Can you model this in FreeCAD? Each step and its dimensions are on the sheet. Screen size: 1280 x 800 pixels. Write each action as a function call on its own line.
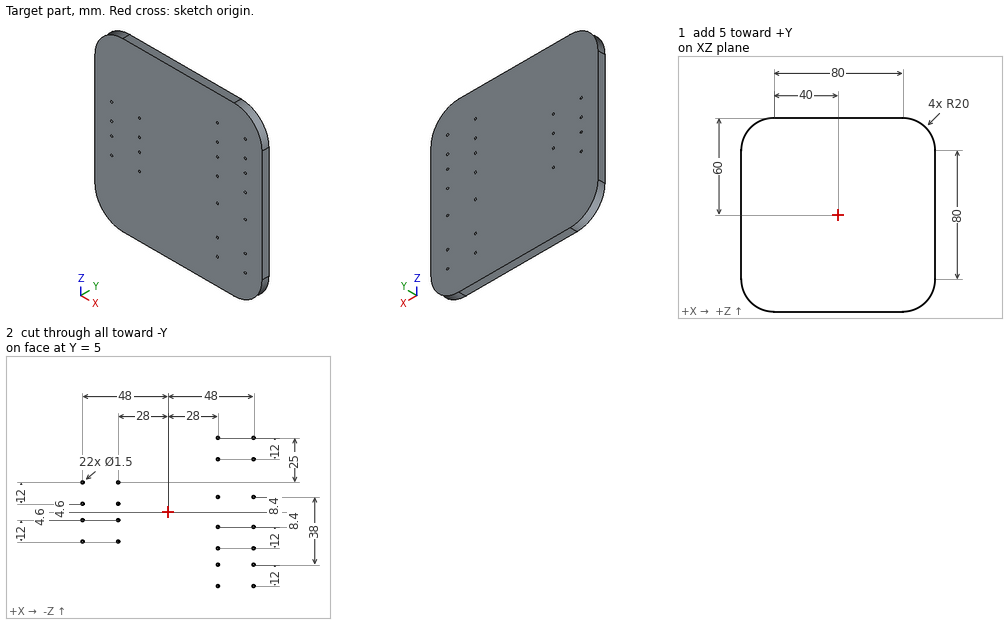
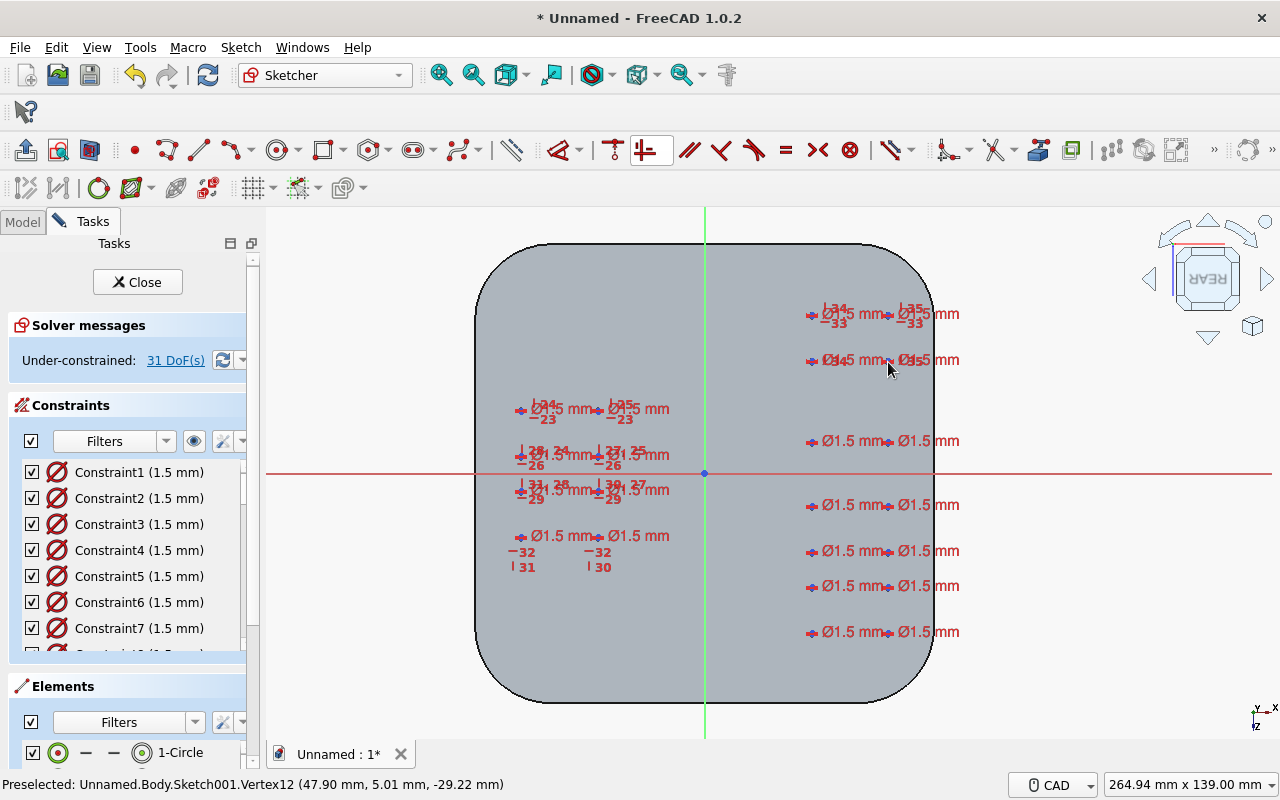
click(812, 362)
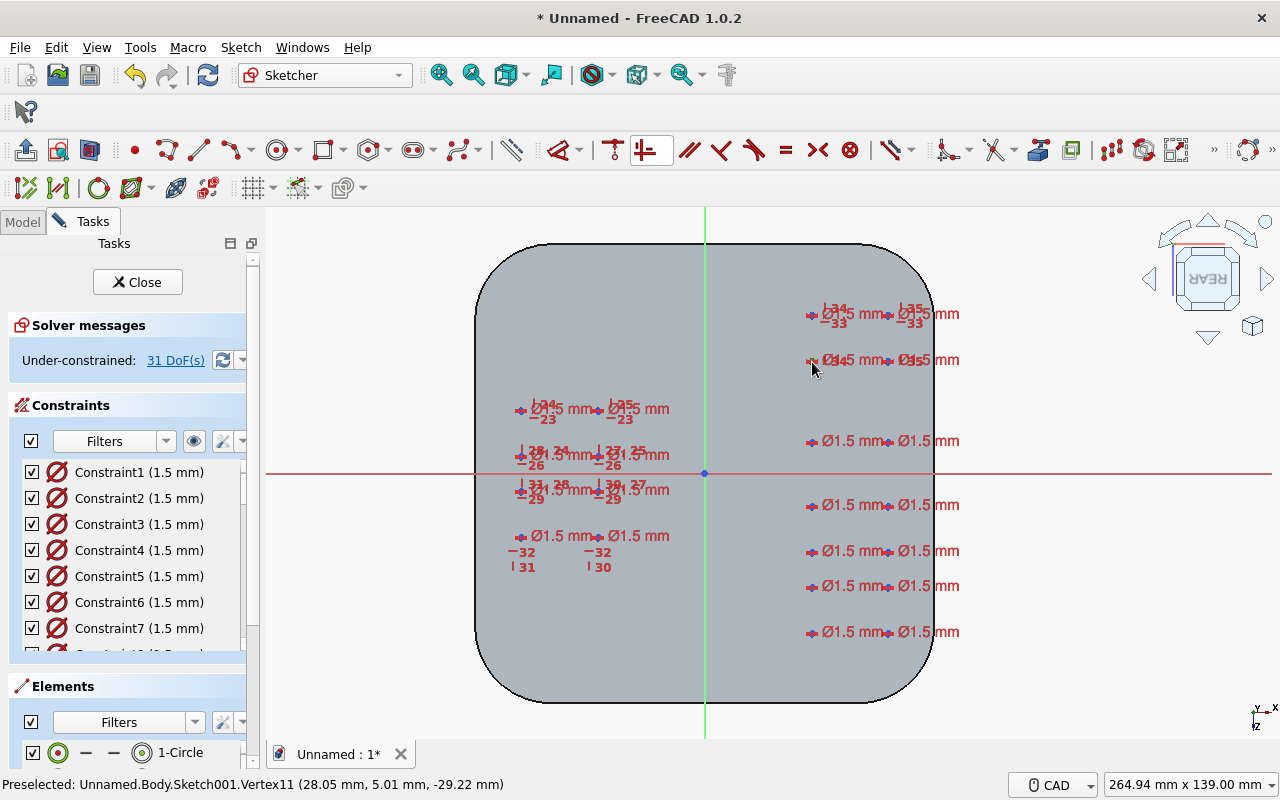
click(888, 362)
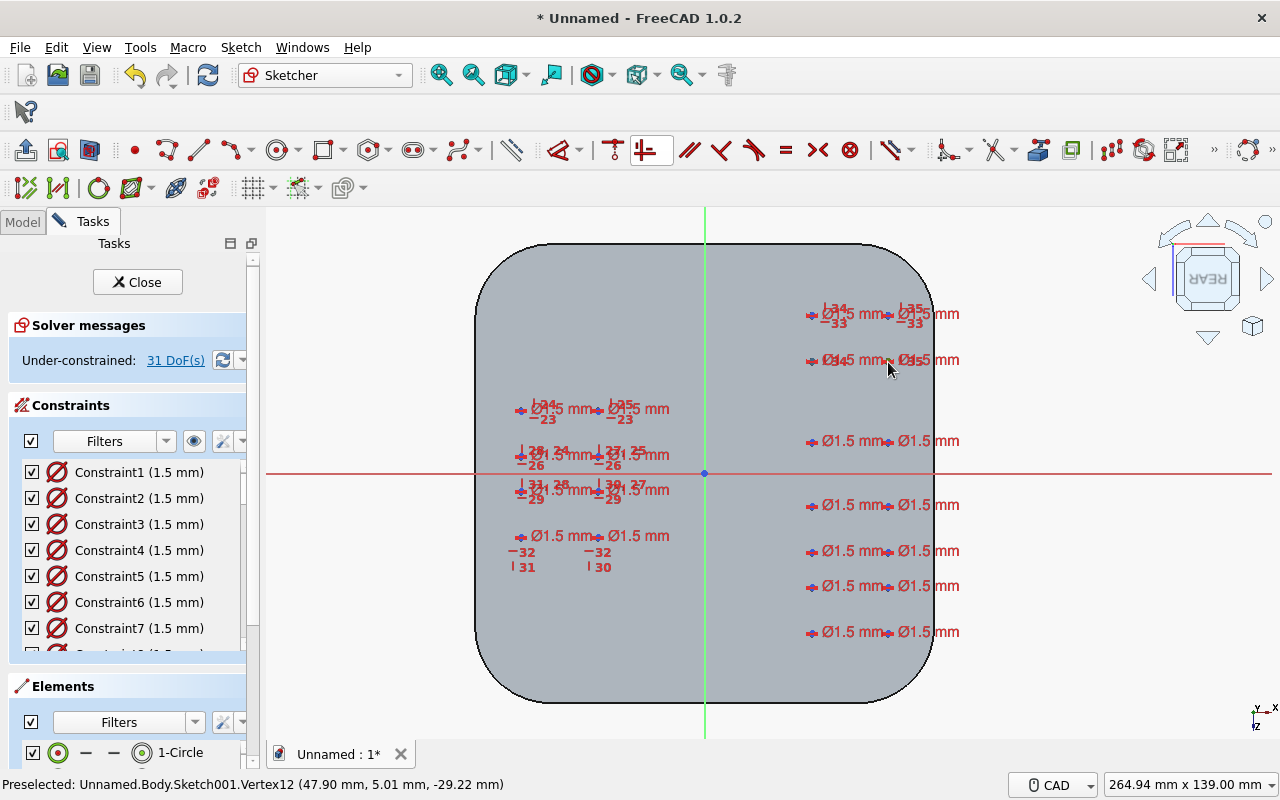
click(668, 150)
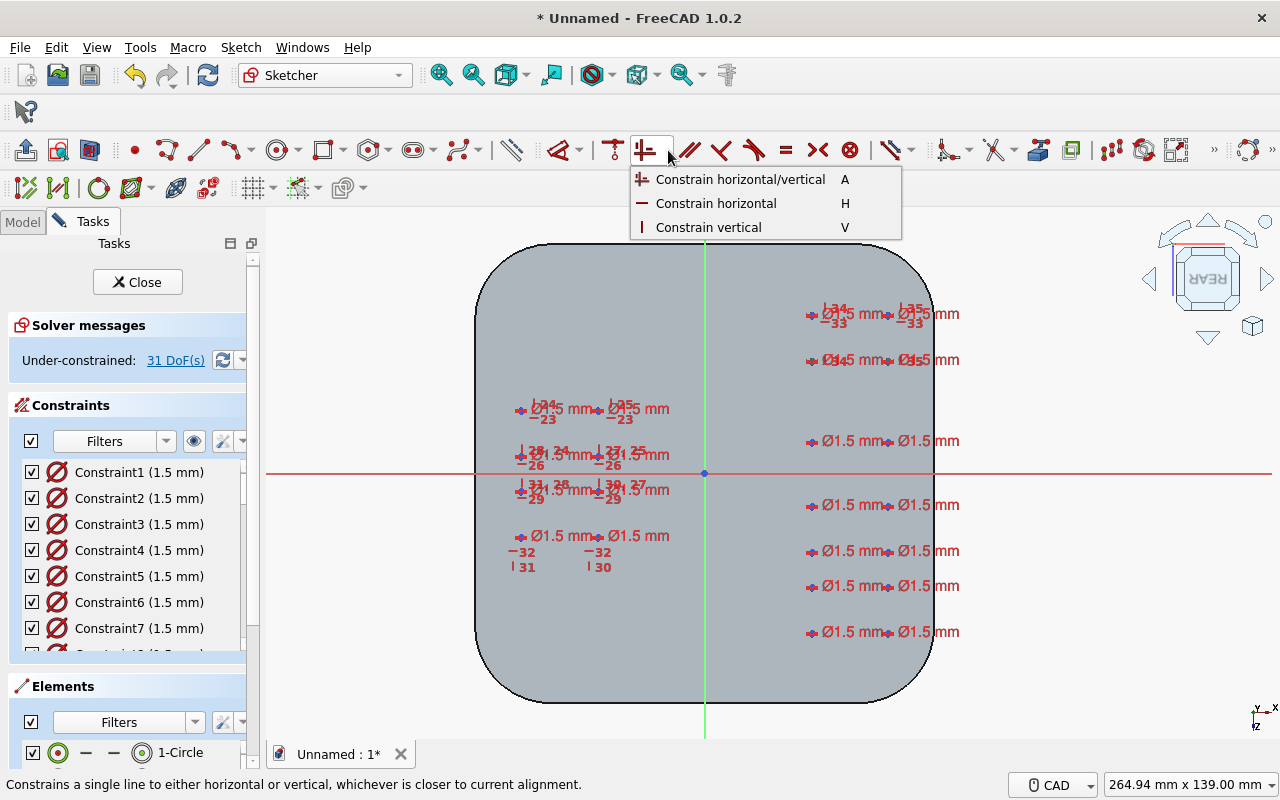
click(766, 203)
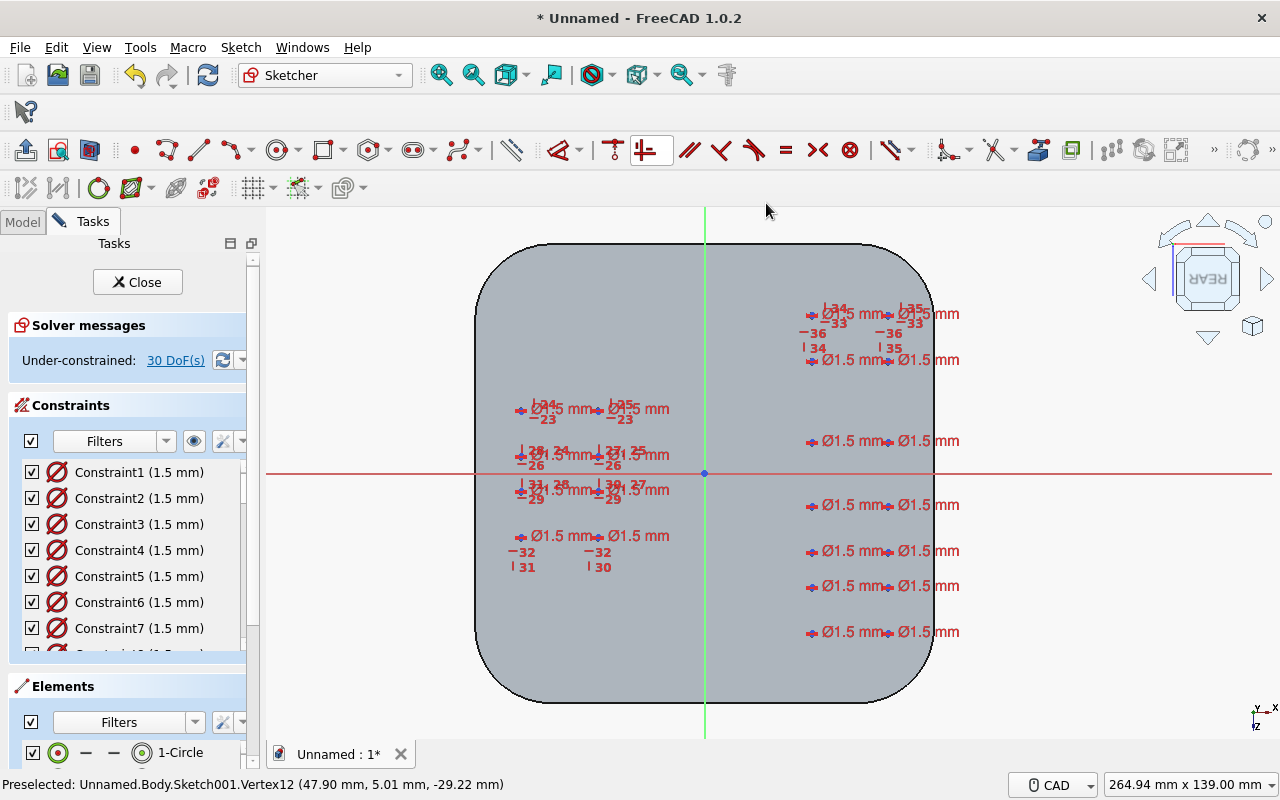
click(888, 362)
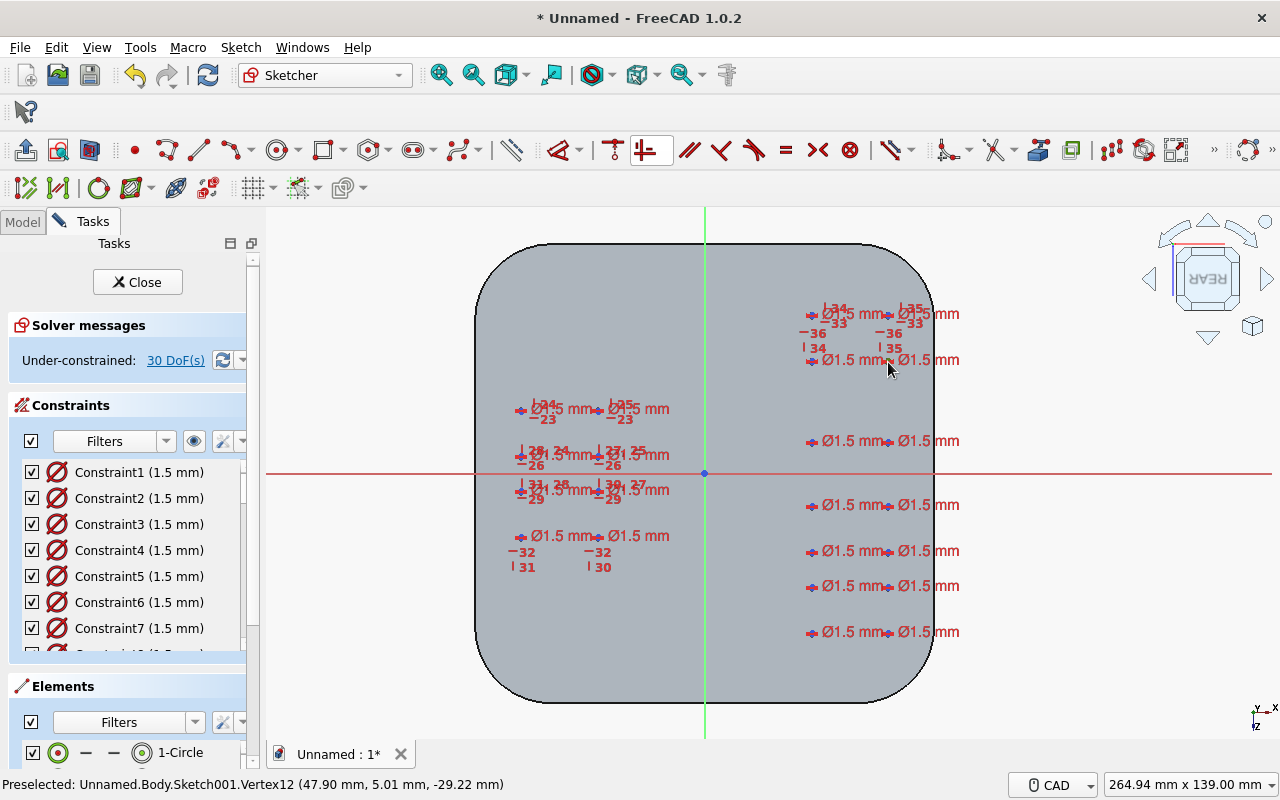
click(888, 443)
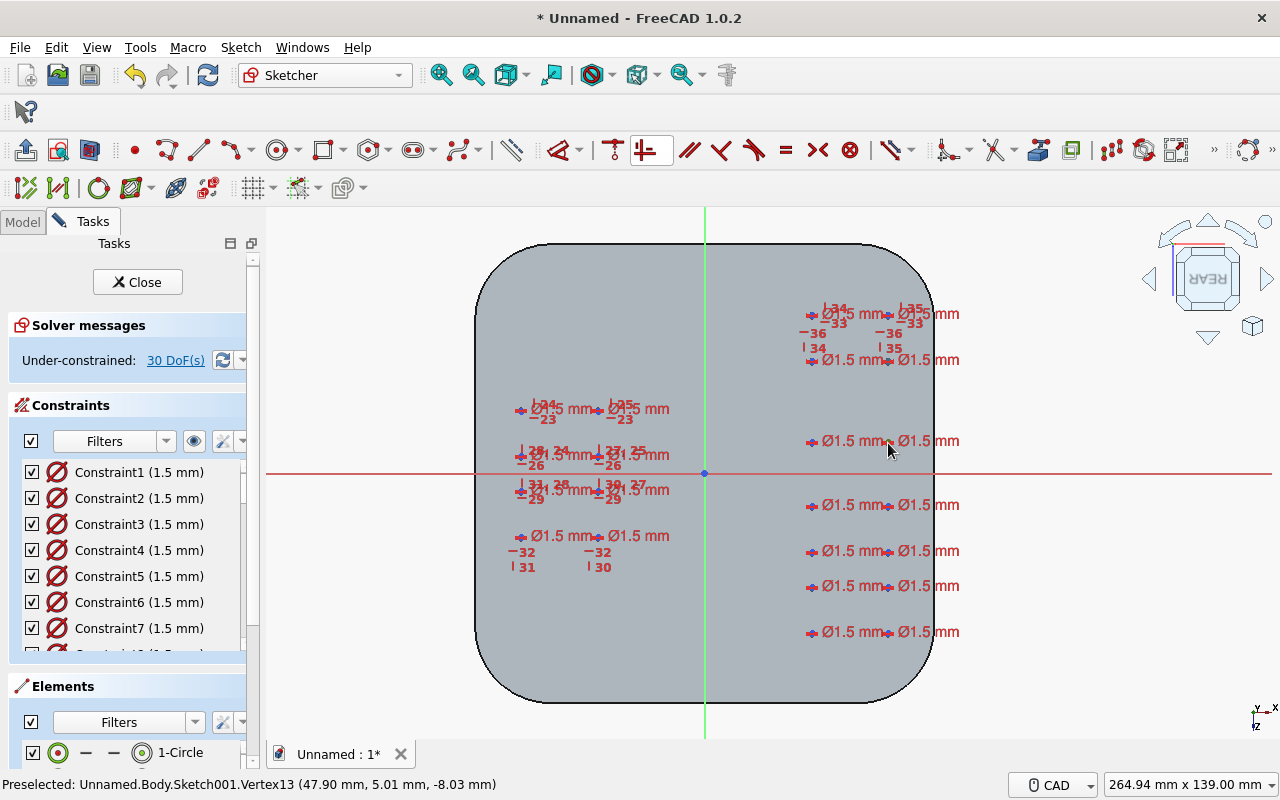
click(668, 150)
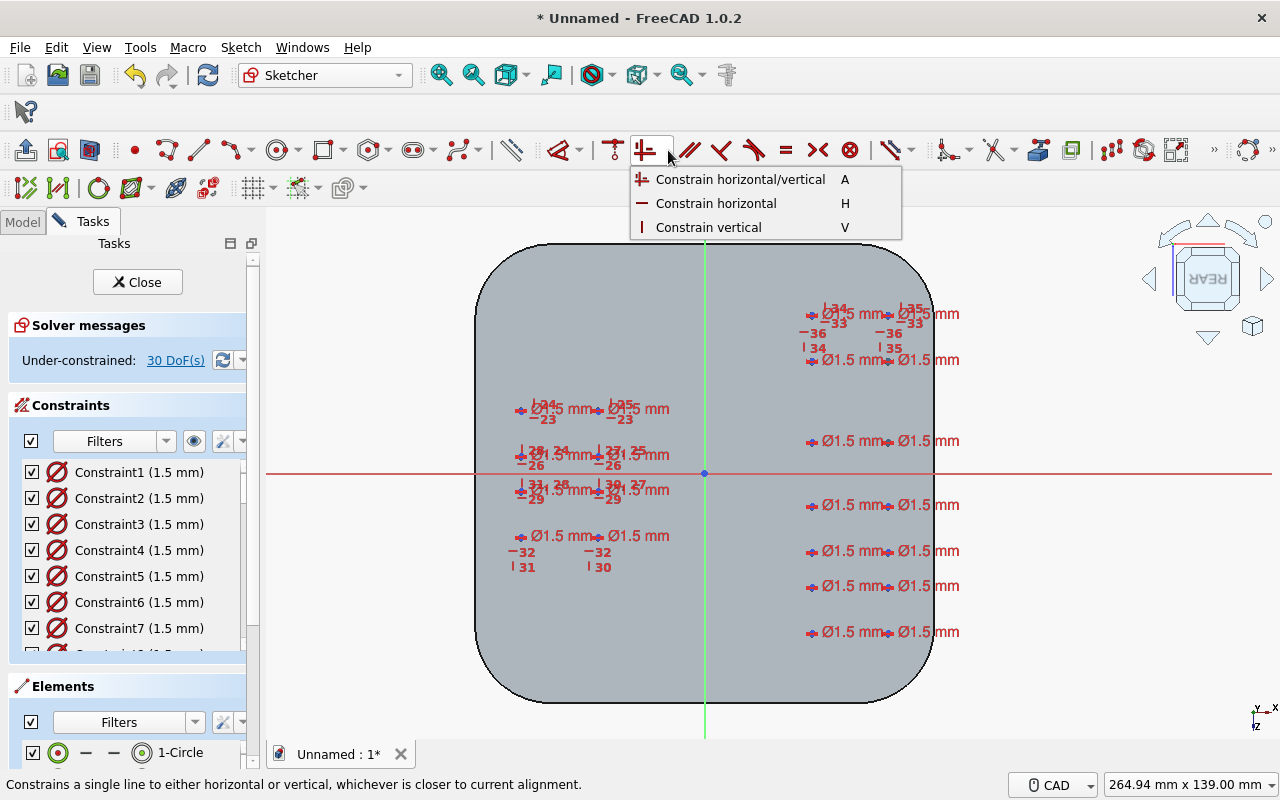
click(766, 227)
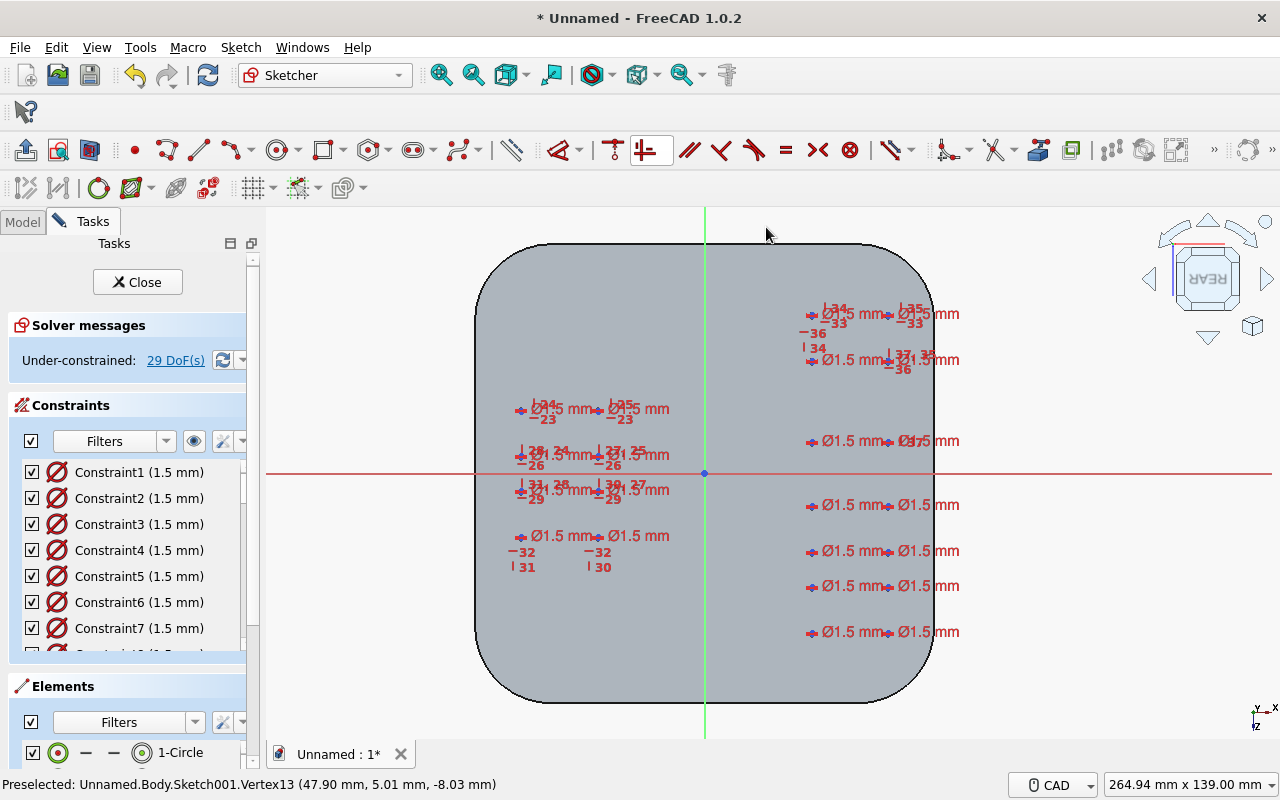
click(812, 362)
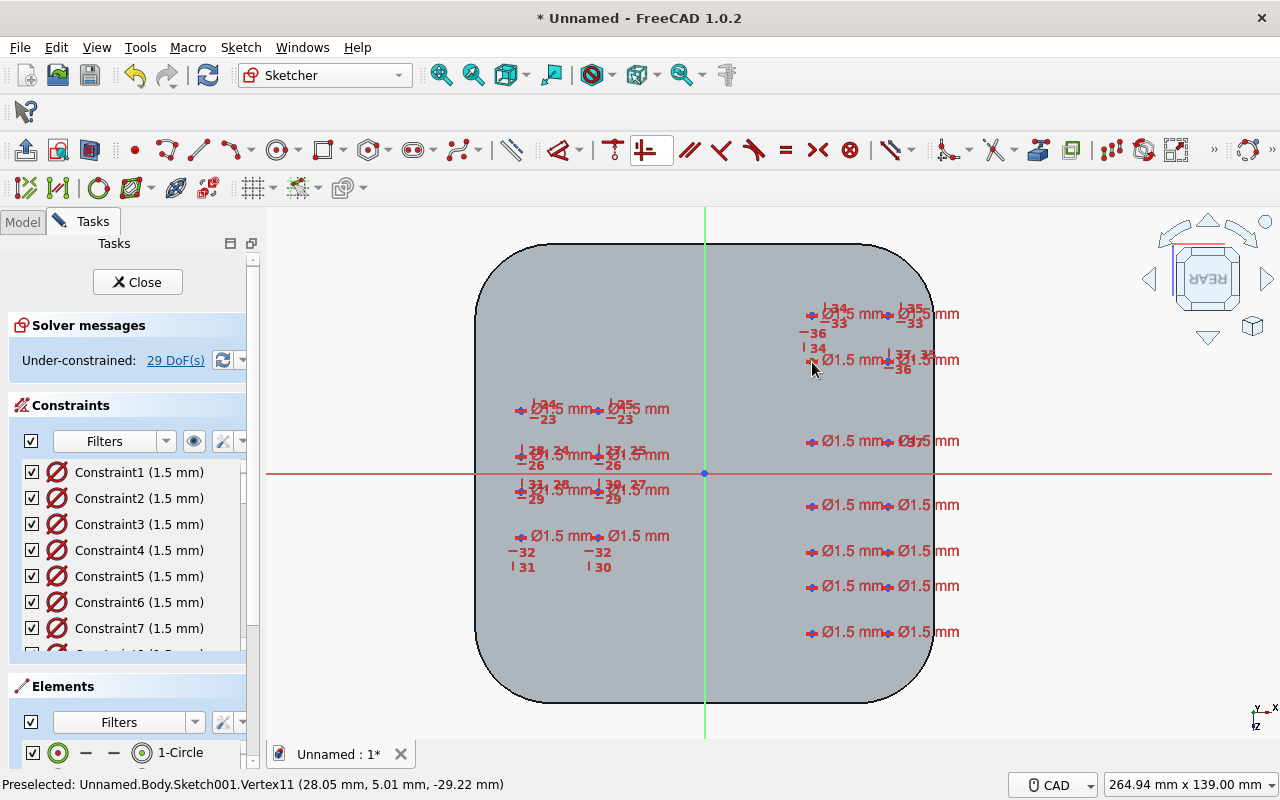
click(812, 443)